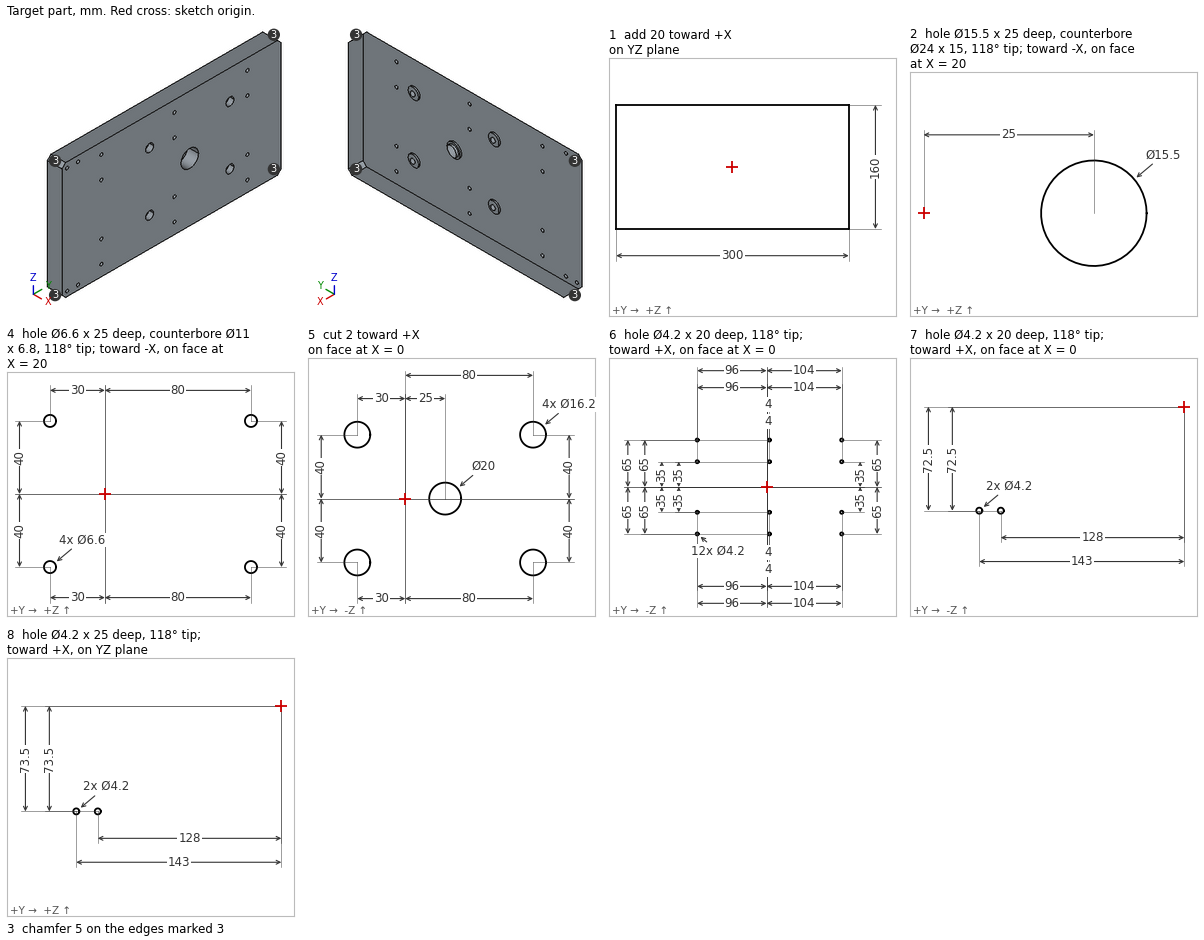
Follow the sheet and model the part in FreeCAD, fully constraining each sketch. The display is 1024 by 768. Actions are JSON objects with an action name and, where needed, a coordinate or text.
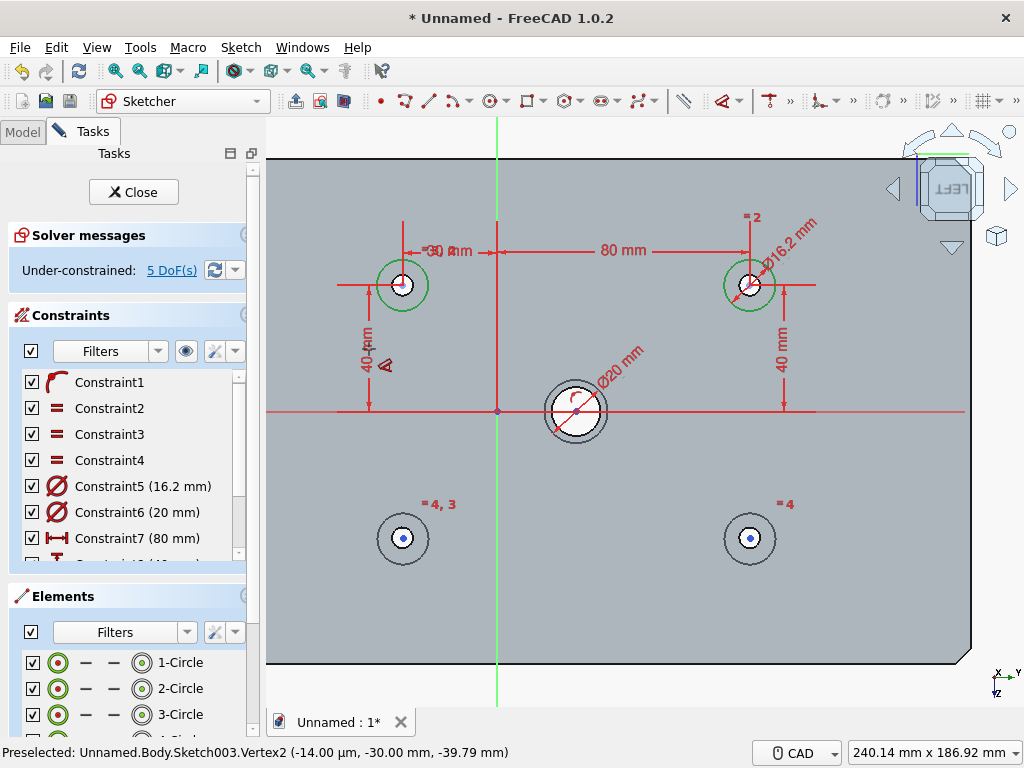
{"action": "left_click", "coordinate": [576, 412]}
{"action": "left_click", "coordinate": [537, 446]}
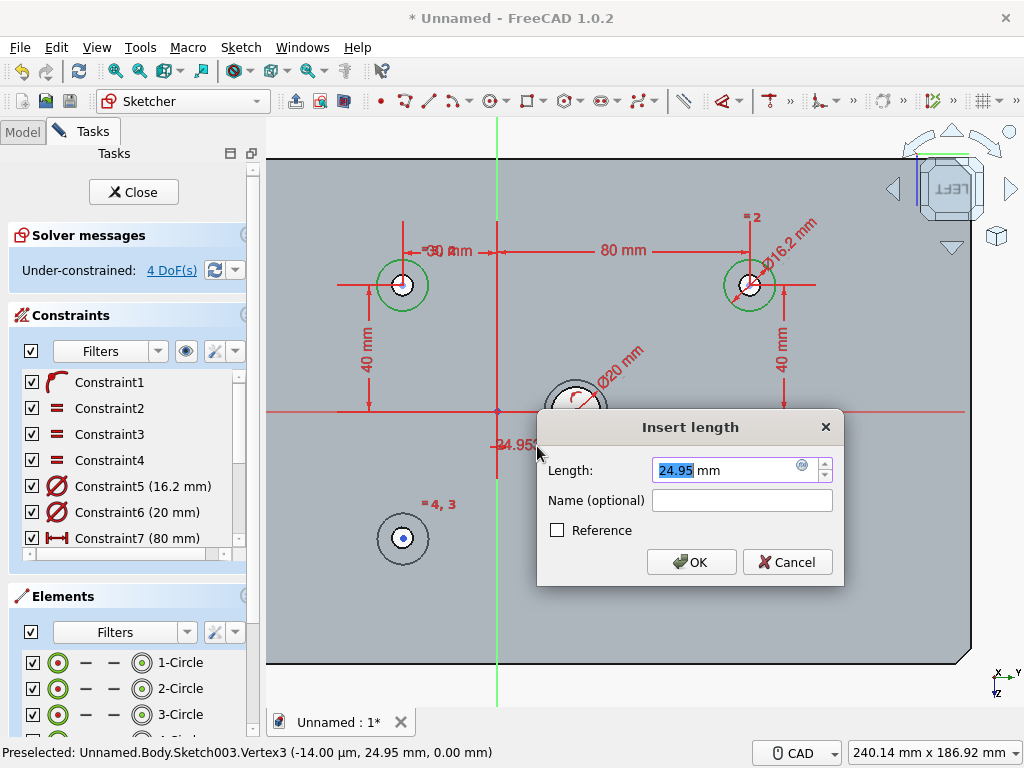
{"action": "type", "text": "25"}
{"action": "key", "text": "Return"}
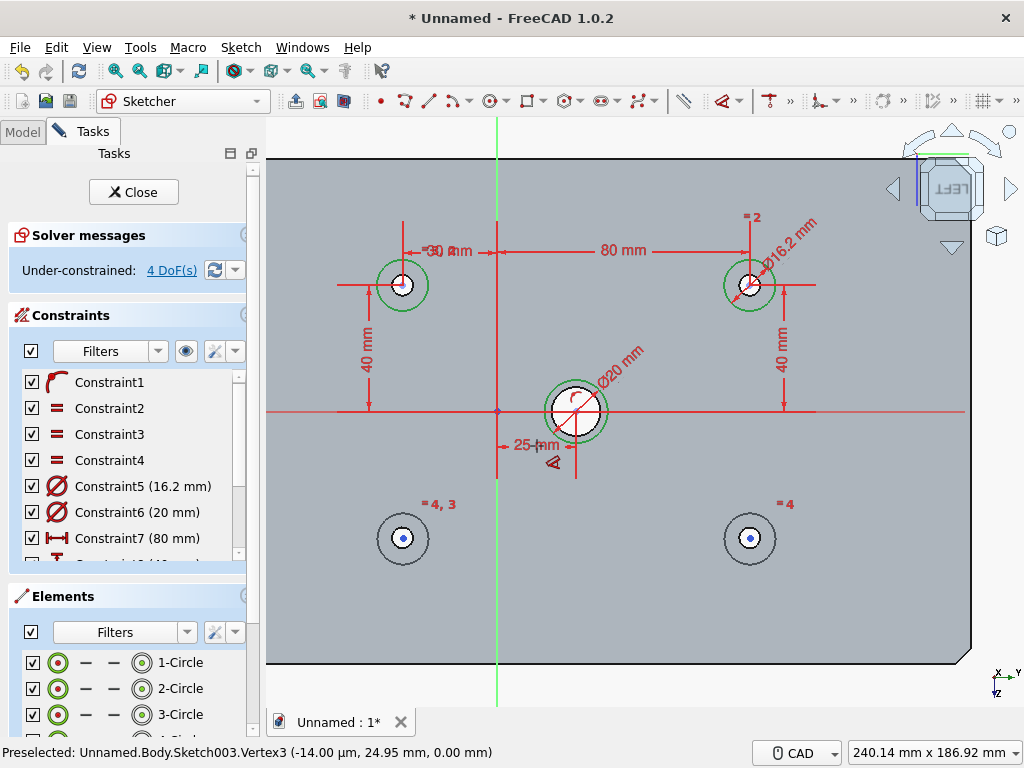
{"action": "left_click", "coordinate": [403, 539]}
{"action": "left_click", "coordinate": [450, 573]}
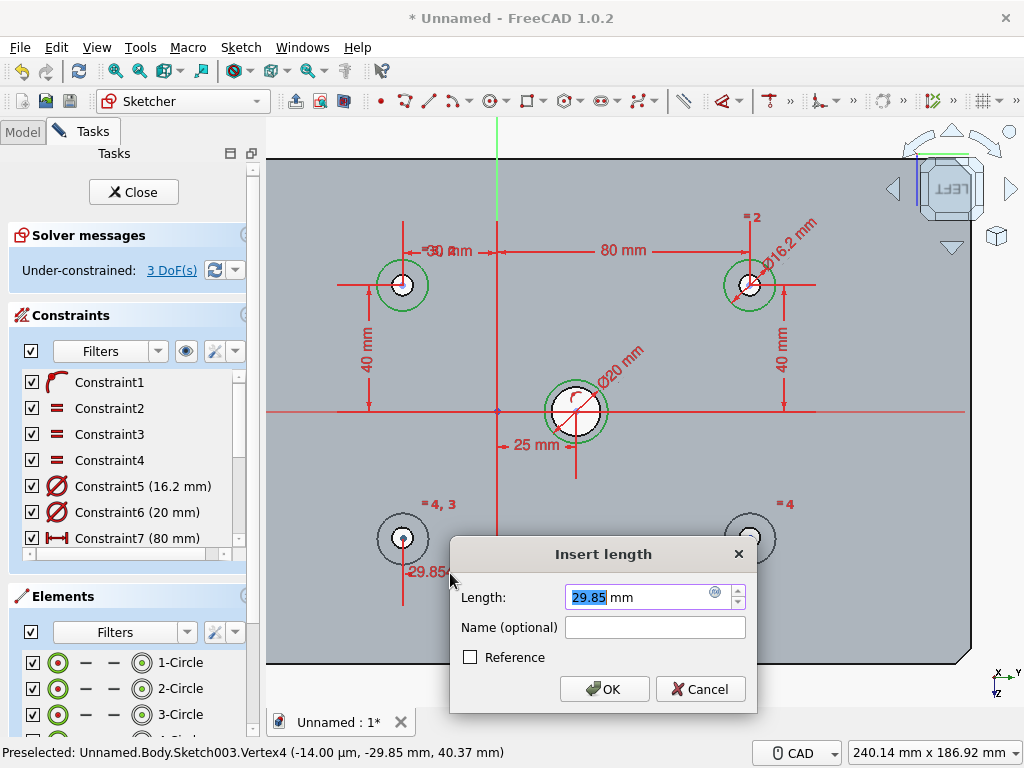
{"action": "type", "text": "30"}
{"action": "key", "text": "Return"}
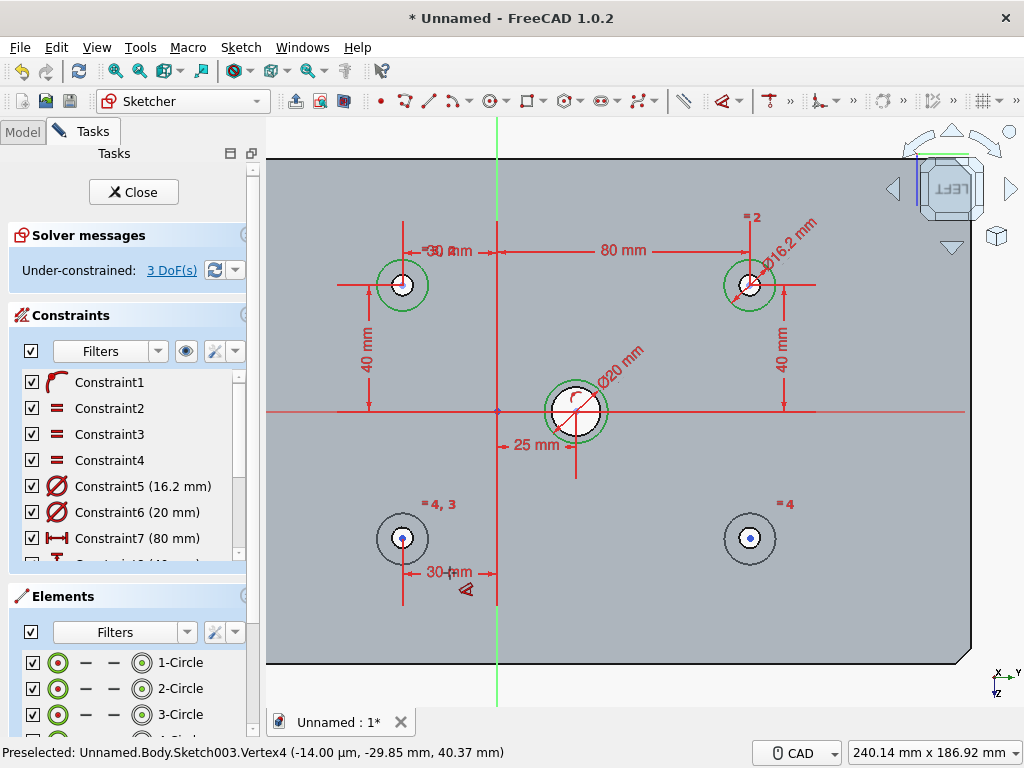
{"action": "left_click", "coordinate": [403, 539]}
{"action": "left_click", "coordinate": [369, 475]}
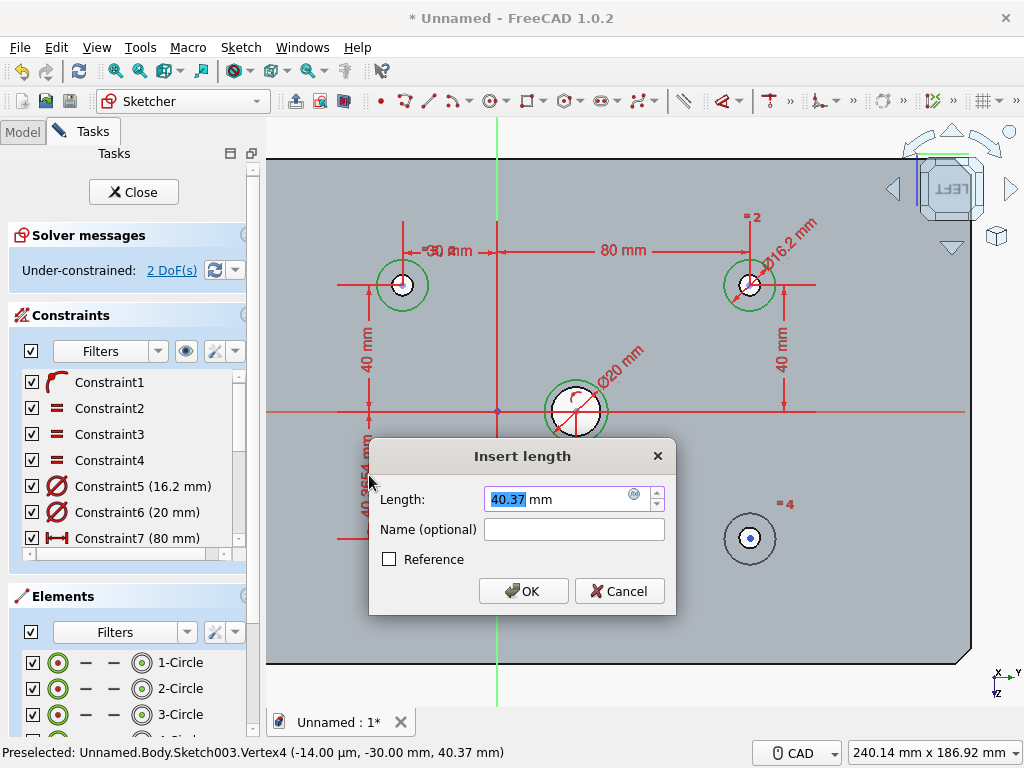
{"action": "type", "text": "40"}
{"action": "key", "text": "Return"}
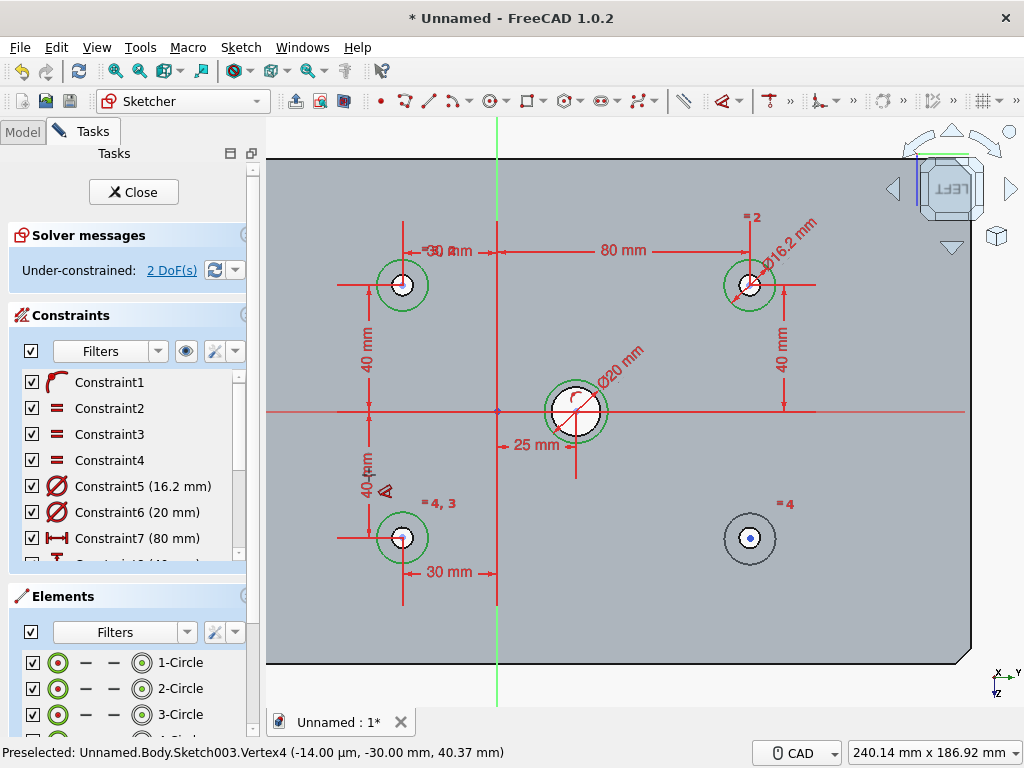
{"action": "left_click", "coordinate": [750, 539]}
{"action": "left_click", "coordinate": [624, 573]}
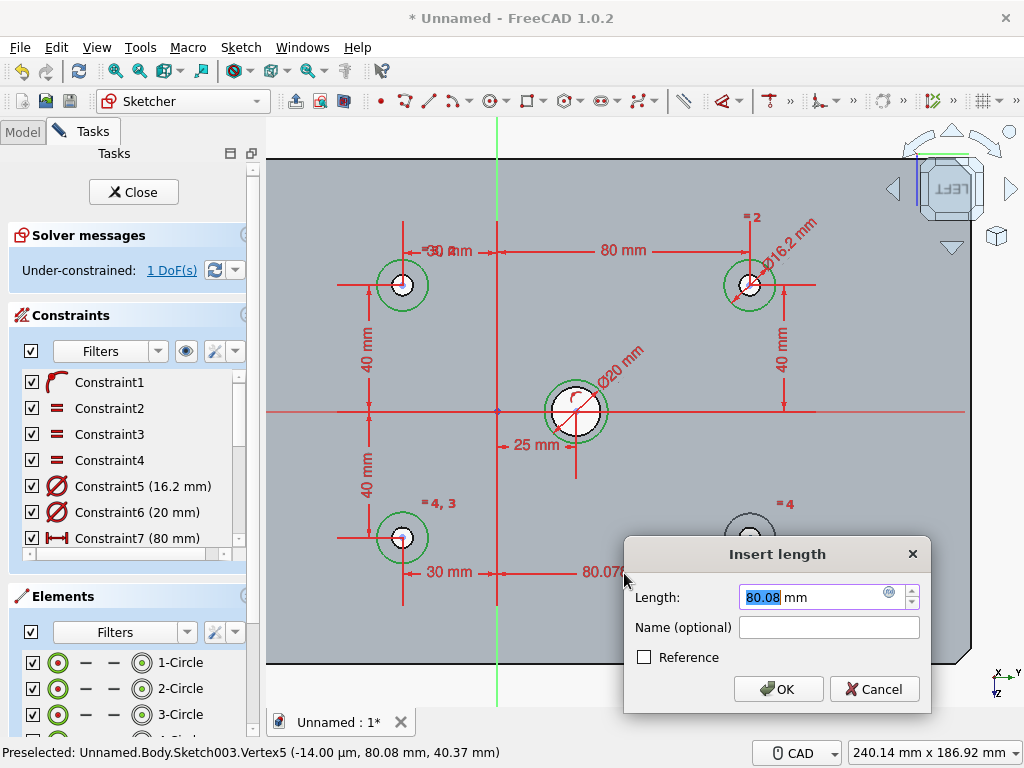
{"action": "type", "text": "80"}
{"action": "key", "text": "Return"}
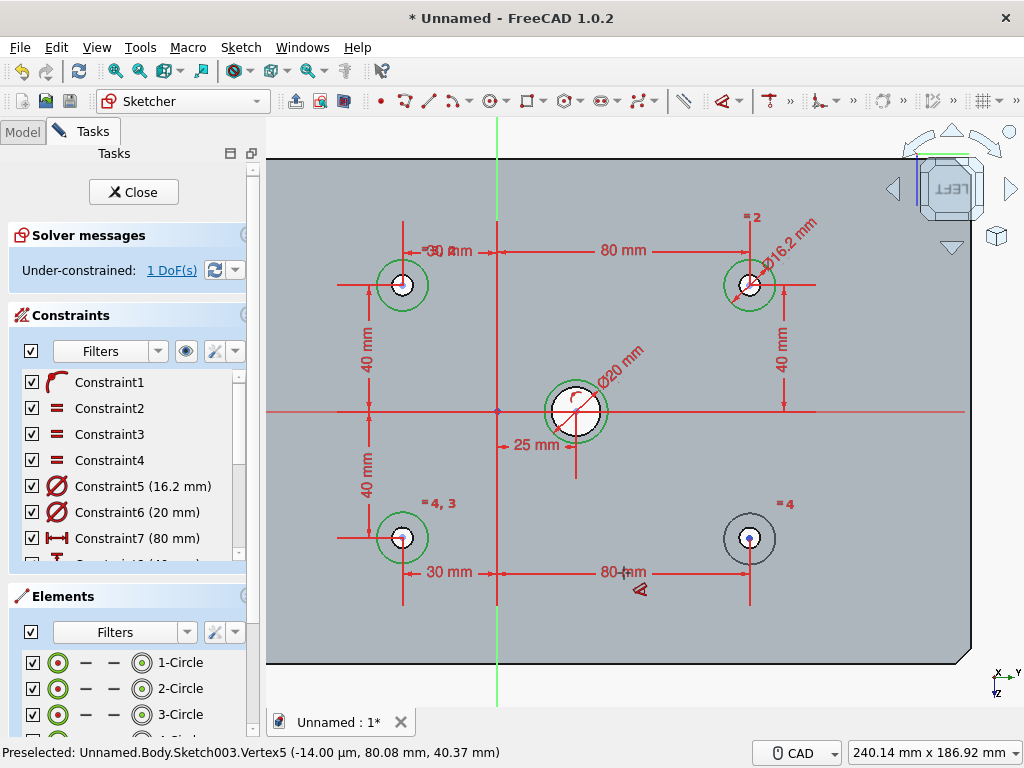
{"action": "left_click", "coordinate": [750, 539]}
{"action": "left_click", "coordinate": [784, 475]}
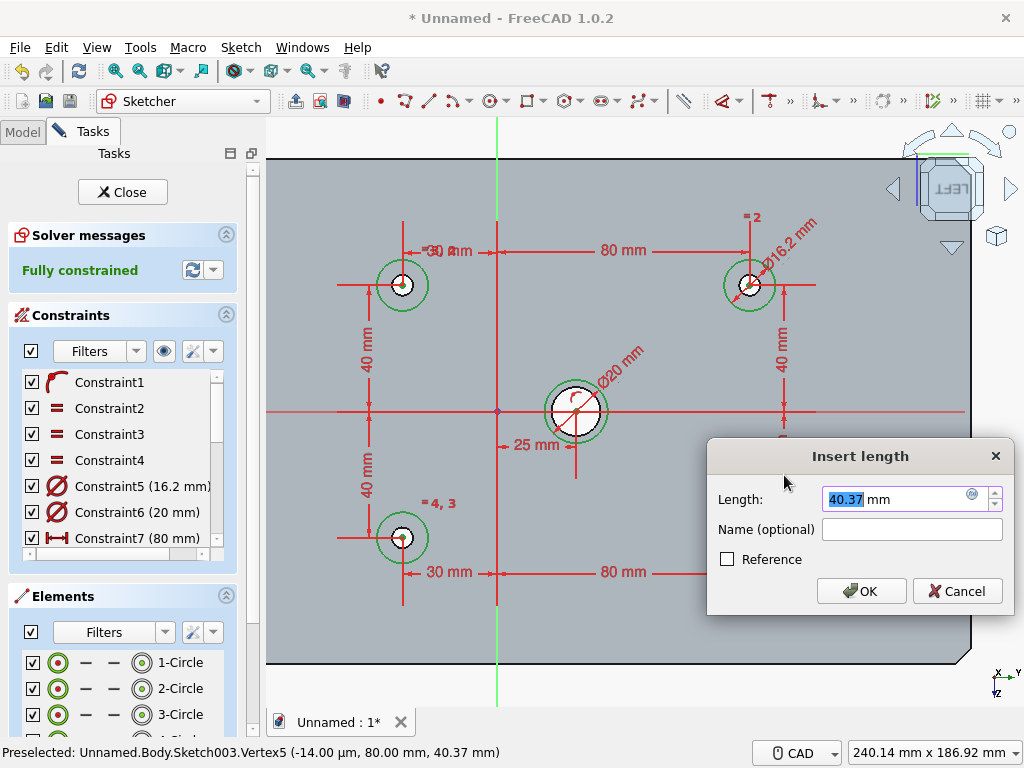
{"action": "type", "text": "40"}
{"action": "key", "text": "Return"}
{"action": "key", "text": "Escape"}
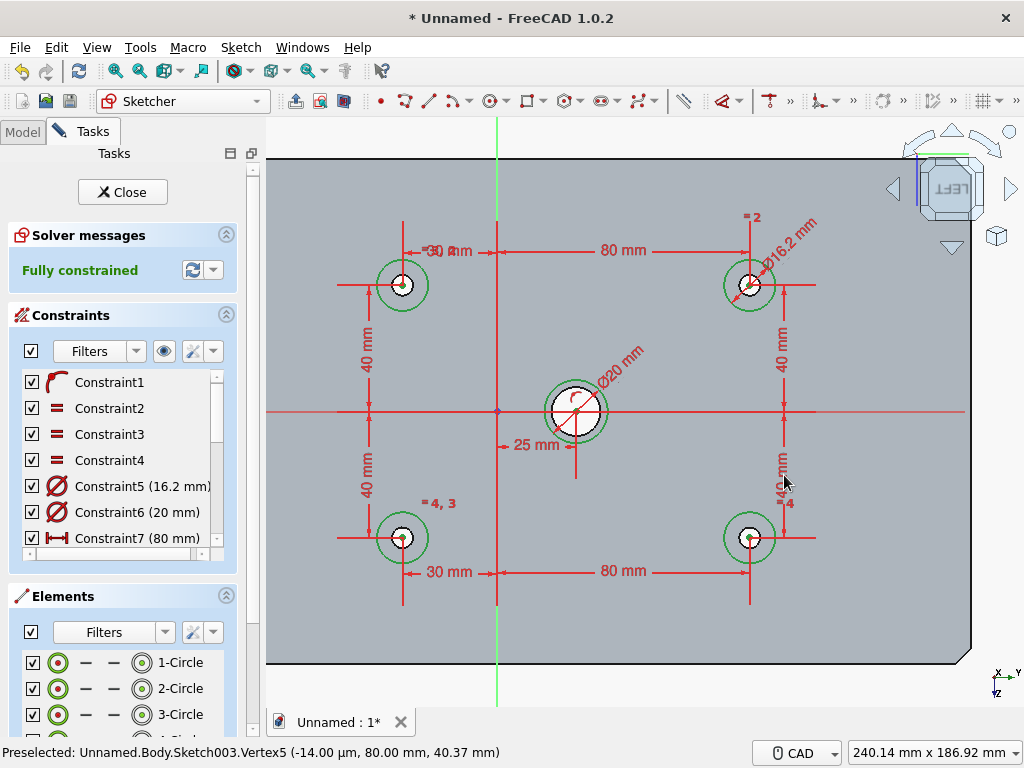
{"action": "left_click", "coordinate": [123, 192]}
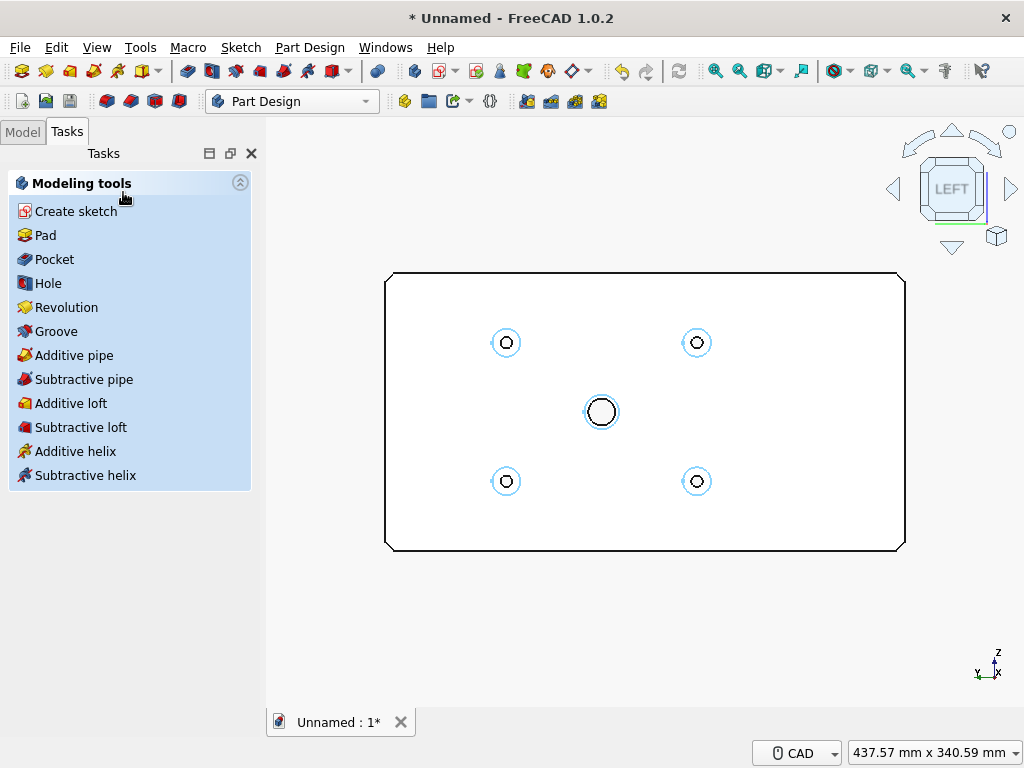
{"action": "left_click", "coordinate": [188, 72]}